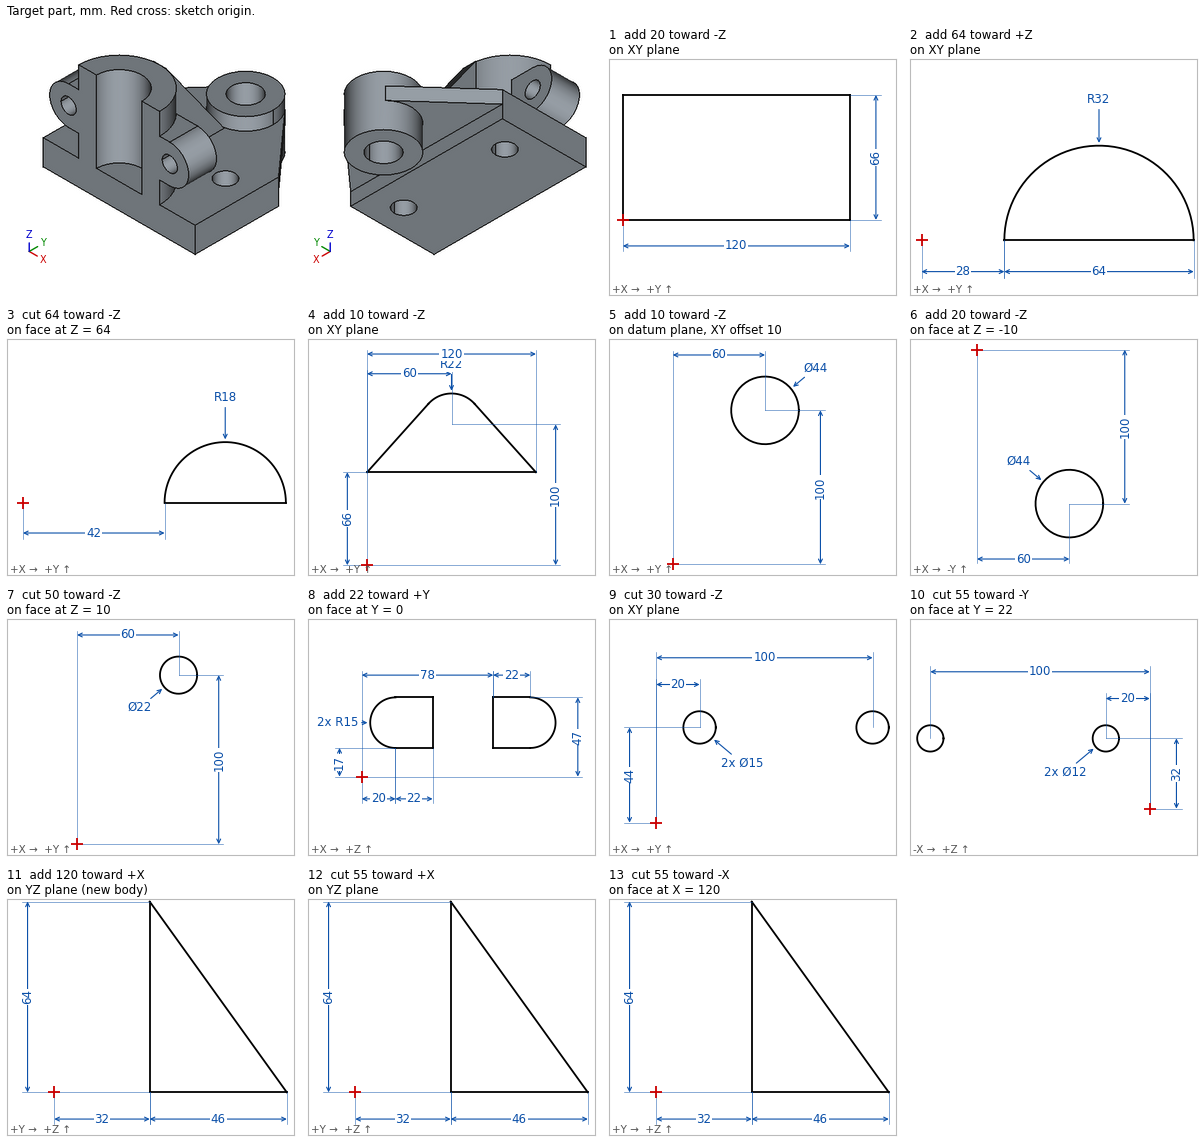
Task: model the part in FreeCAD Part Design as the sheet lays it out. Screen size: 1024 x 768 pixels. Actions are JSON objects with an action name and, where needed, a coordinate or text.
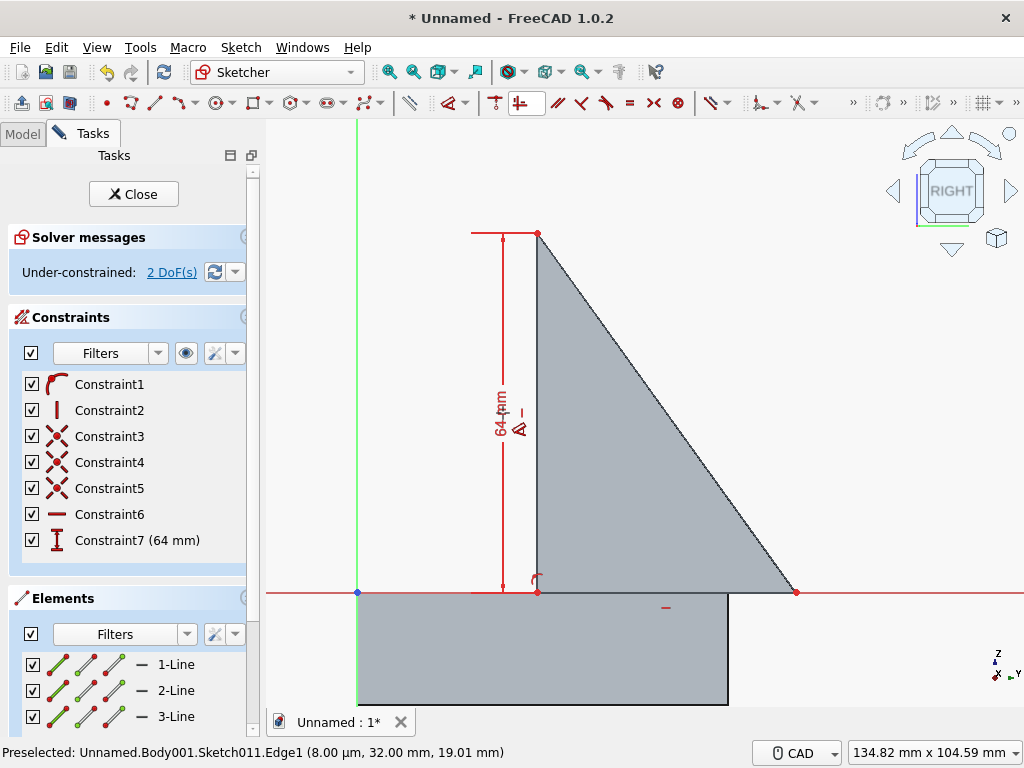
{"action": "left_click", "coordinate": [718, 593]}
{"action": "left_click", "coordinate": [666, 627]}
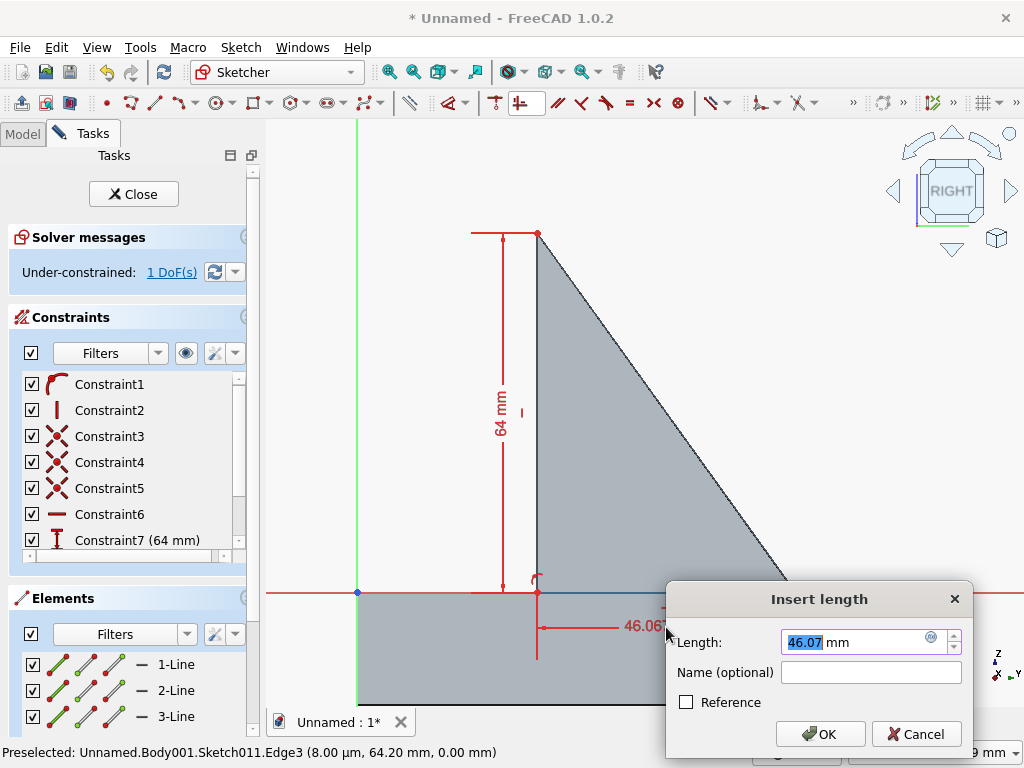
{"action": "type", "text": "46"}
{"action": "key", "text": "Return"}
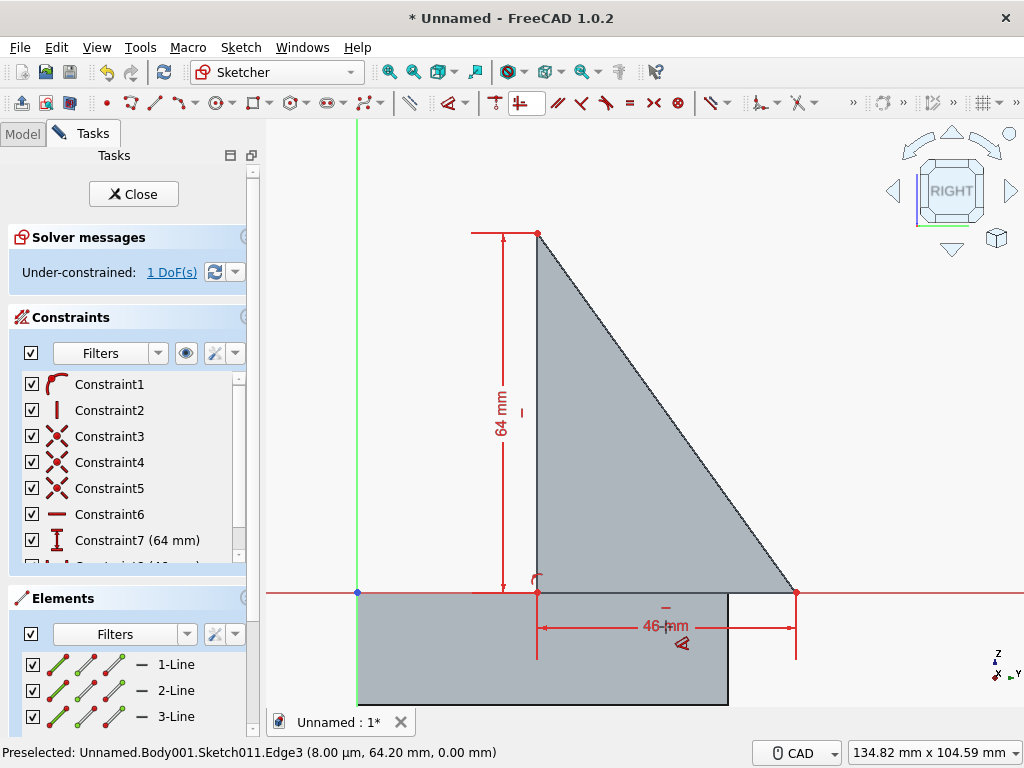
{"action": "left_click", "coordinate": [537, 593]}
{"action": "left_click", "coordinate": [447, 627]}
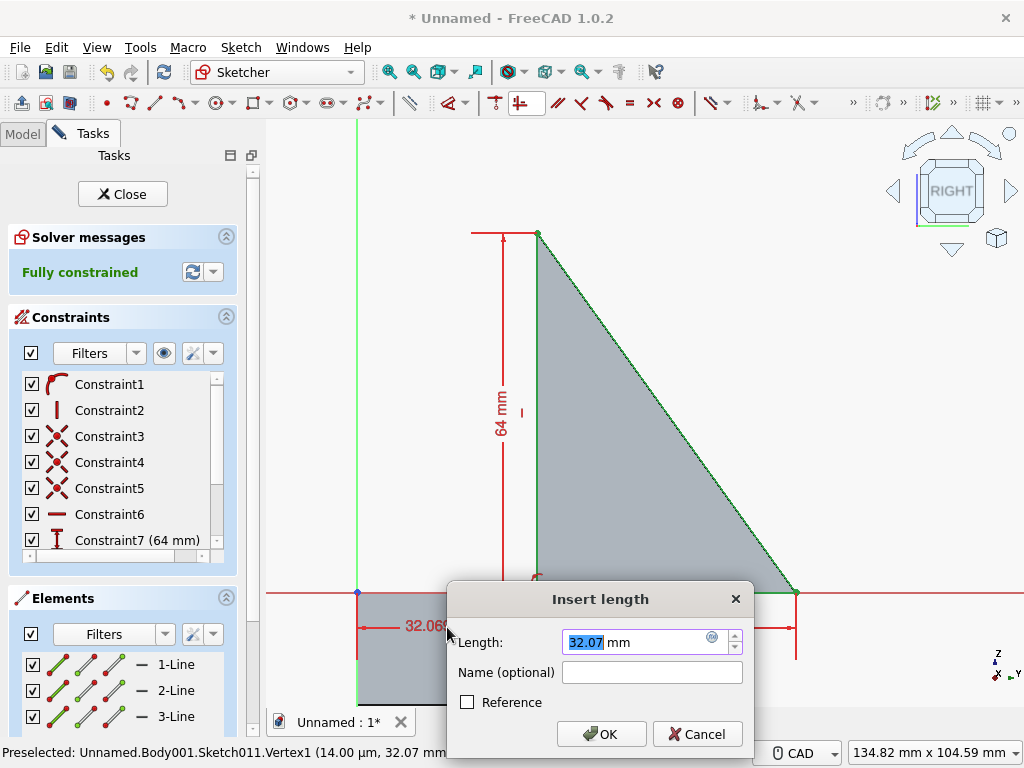
{"action": "type", "text": "32"}
{"action": "key", "text": "Return"}
{"action": "key", "text": "Escape"}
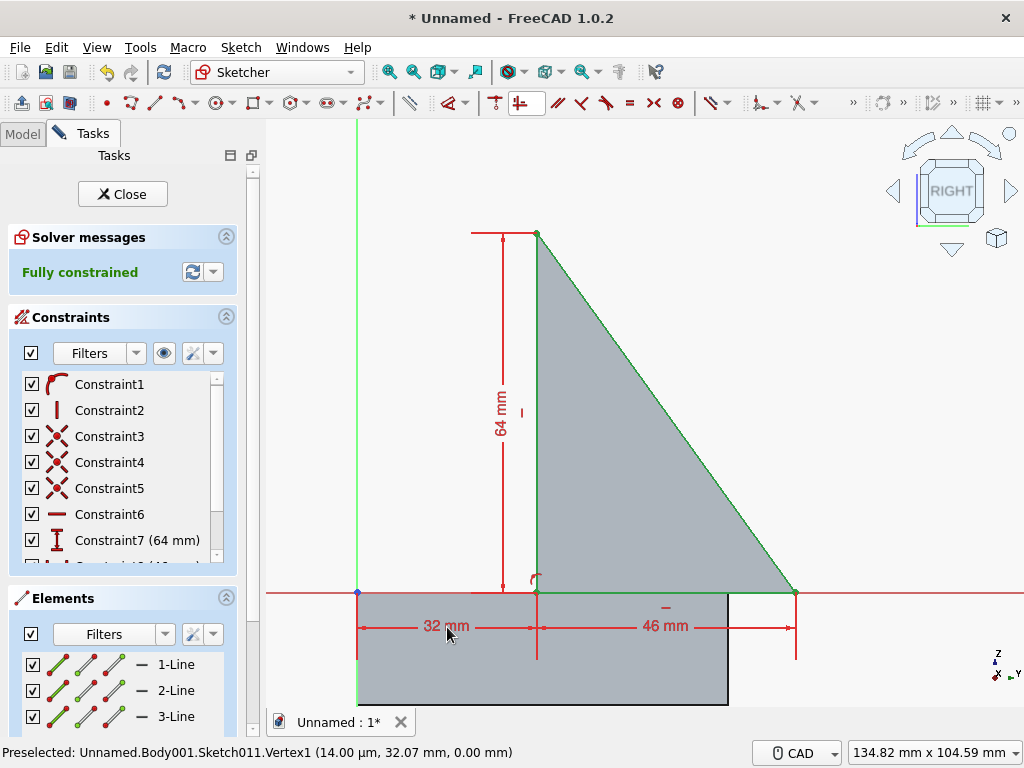
{"action": "left_click", "coordinate": [123, 194]}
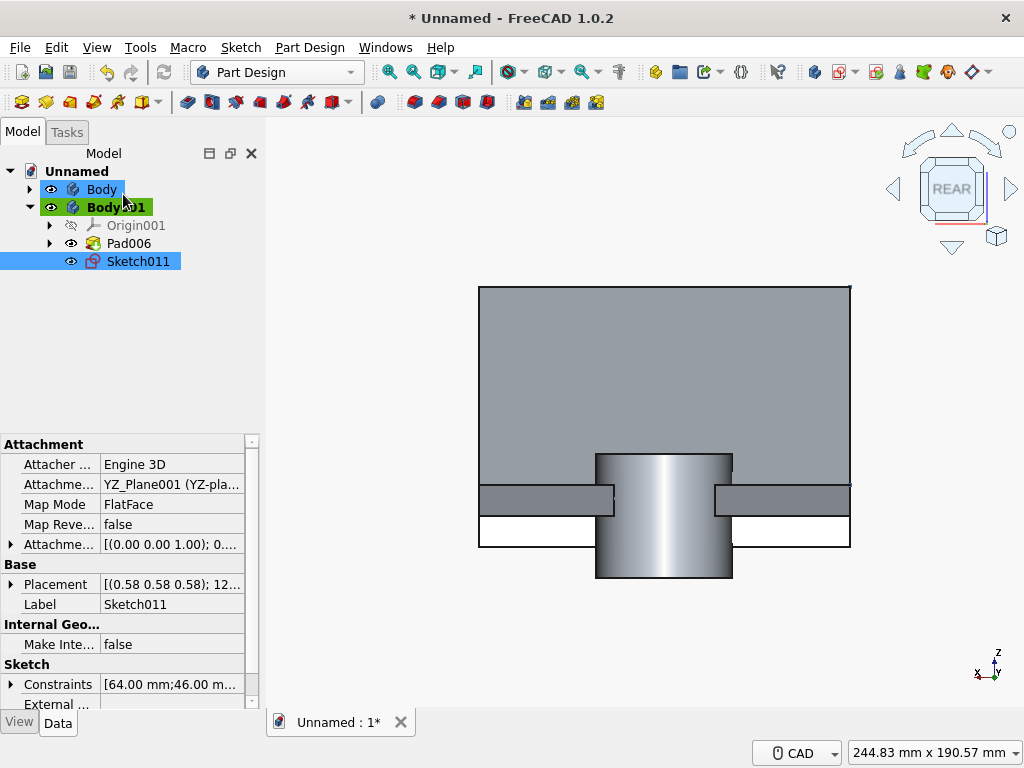
{"action": "left_click", "coordinate": [188, 102]}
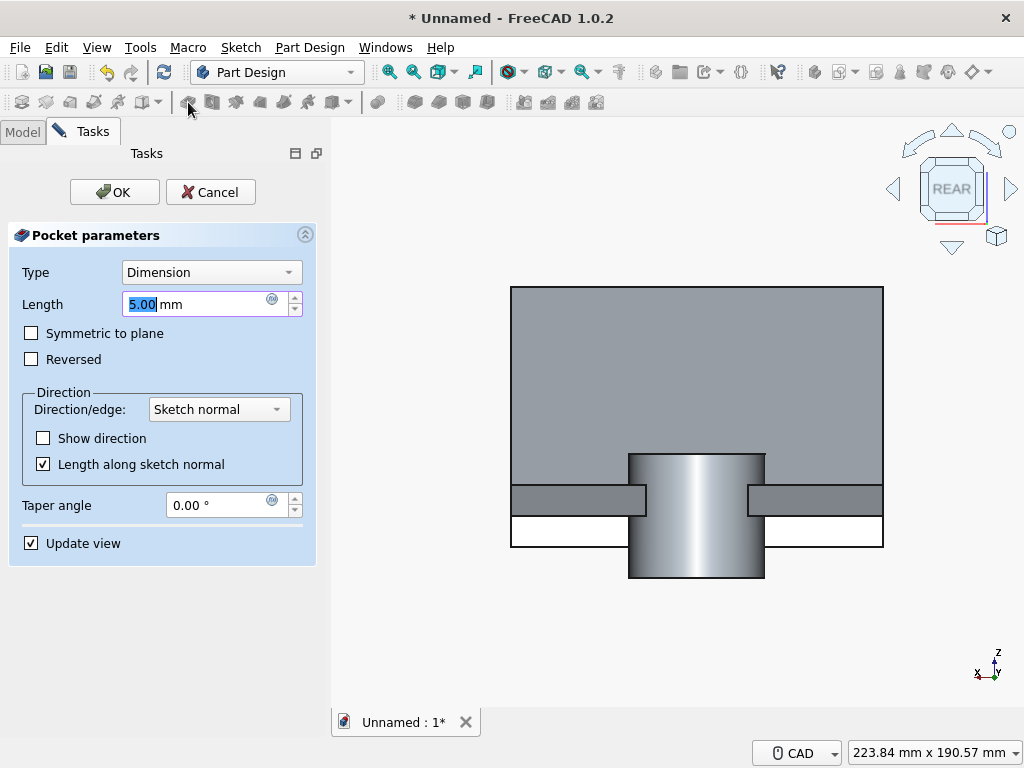
{"action": "type", "text": "55"}
{"action": "key", "text": "Tab"}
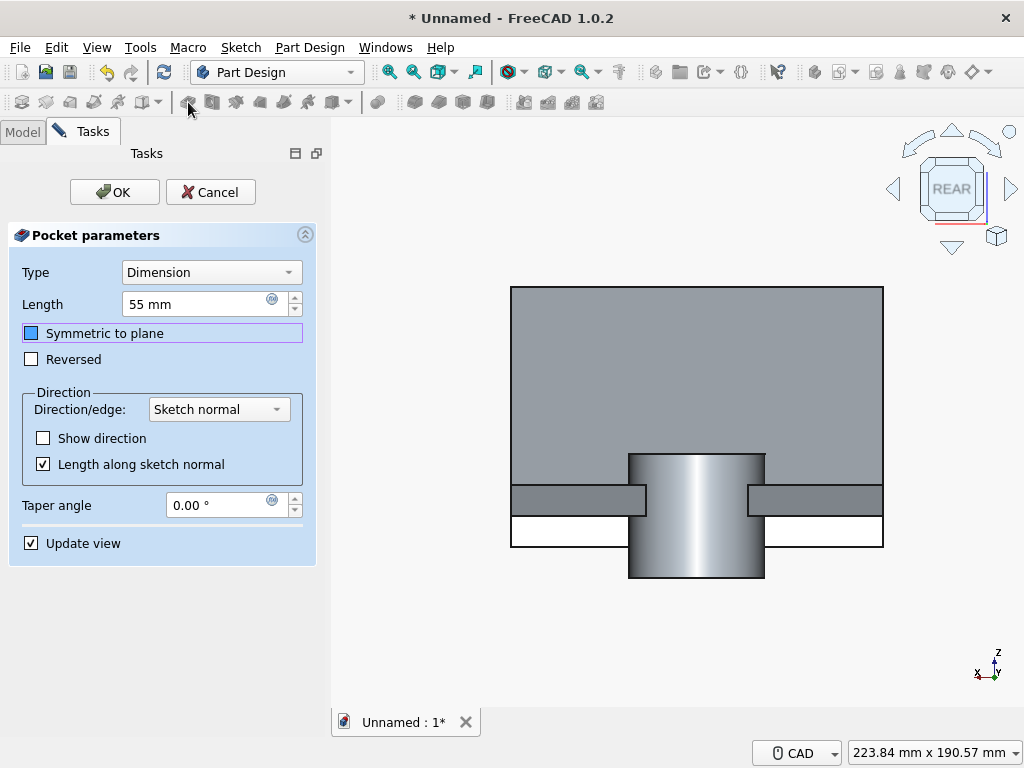
{"action": "left_click", "coordinate": [30, 359]}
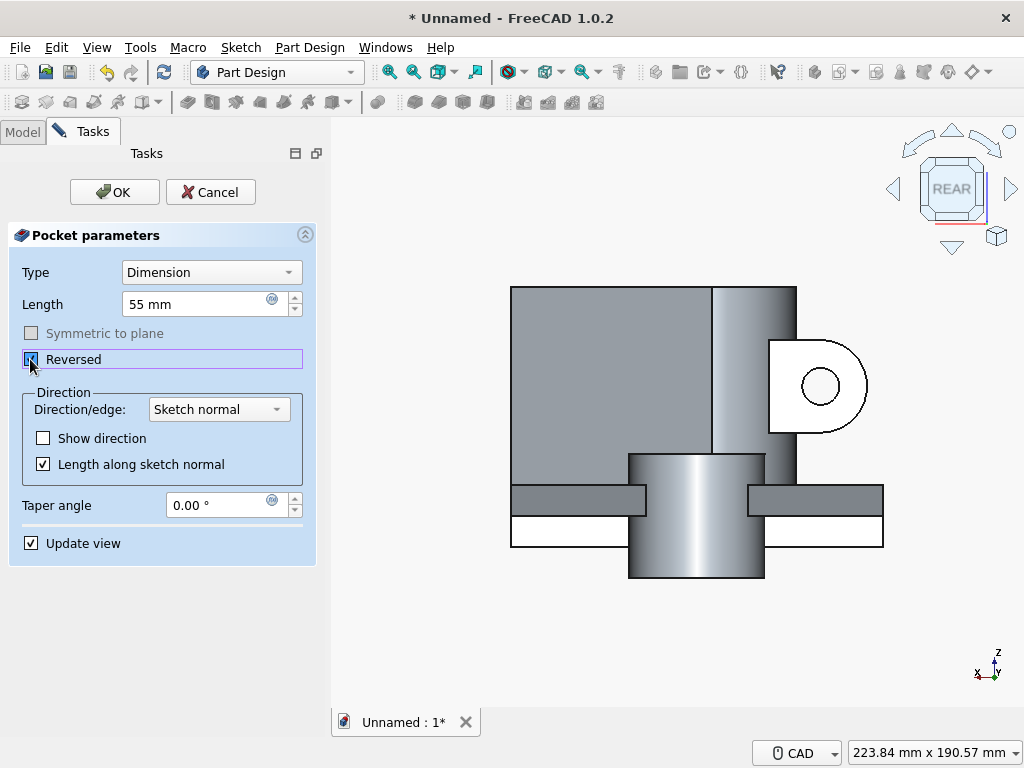
{"action": "left_click", "coordinate": [115, 192]}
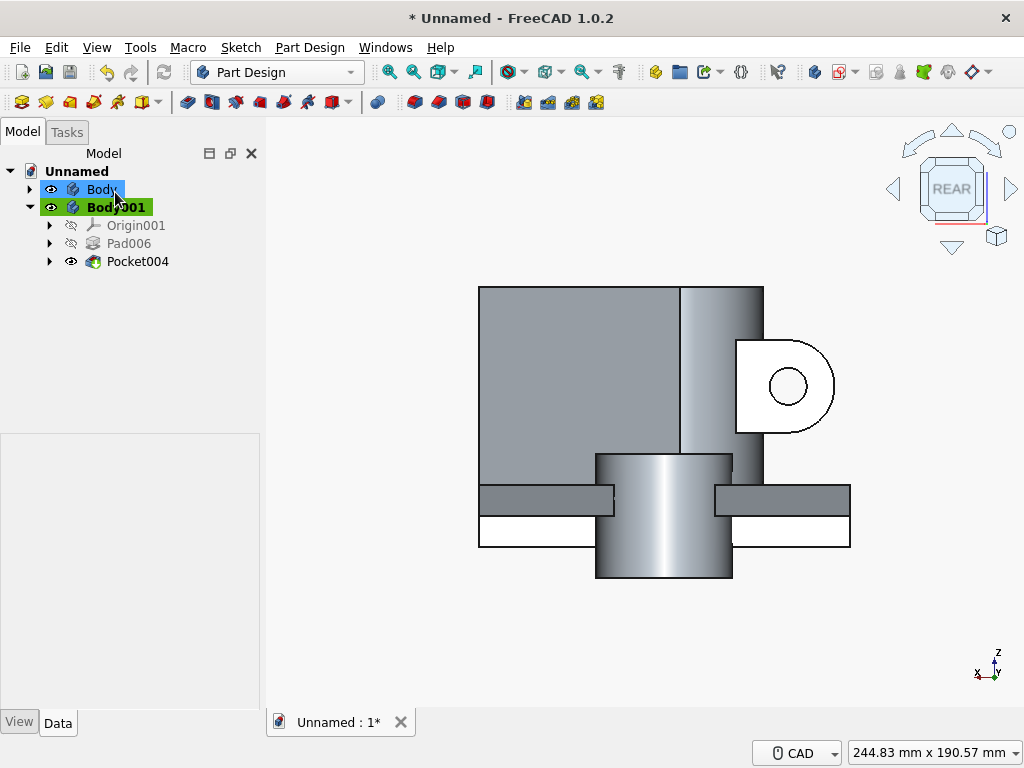
{"action": "left_click", "coordinate": [390, 72]}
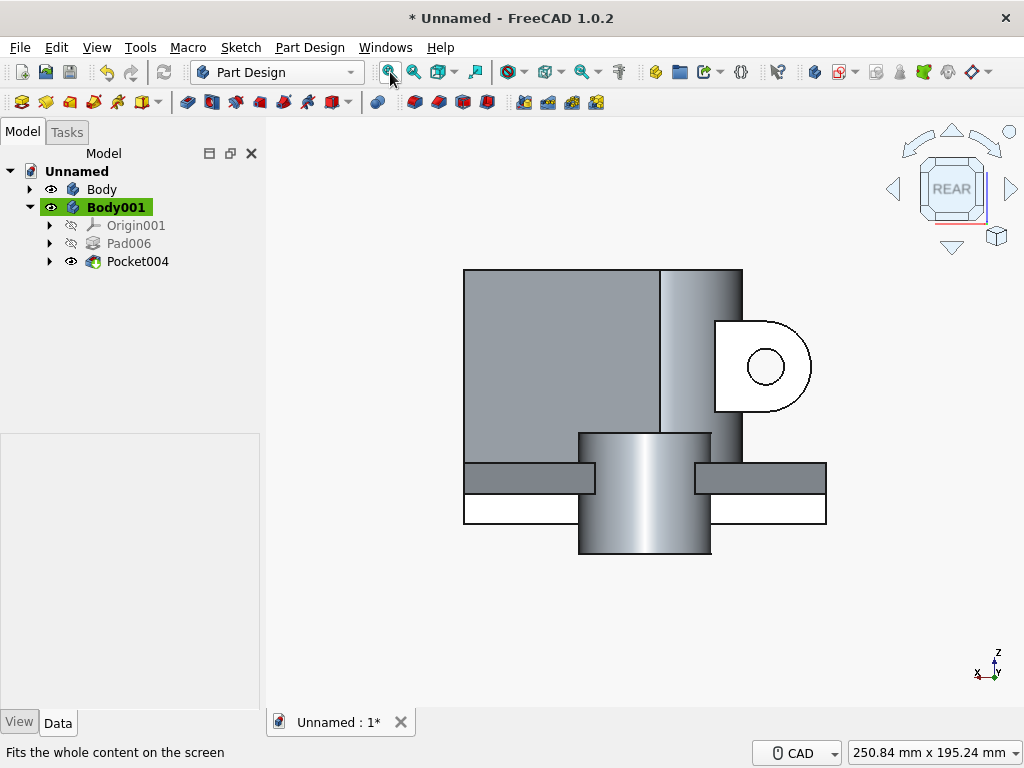
{"action": "key", "text": "0"}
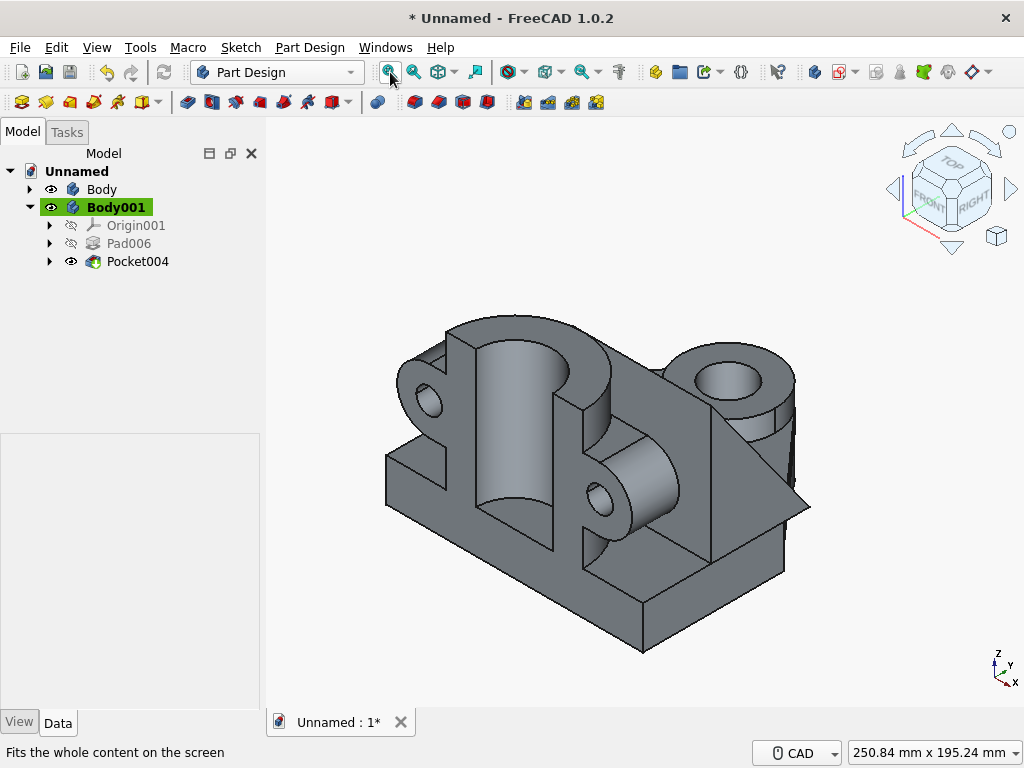
{"action": "left_click", "coordinate": [746, 509]}